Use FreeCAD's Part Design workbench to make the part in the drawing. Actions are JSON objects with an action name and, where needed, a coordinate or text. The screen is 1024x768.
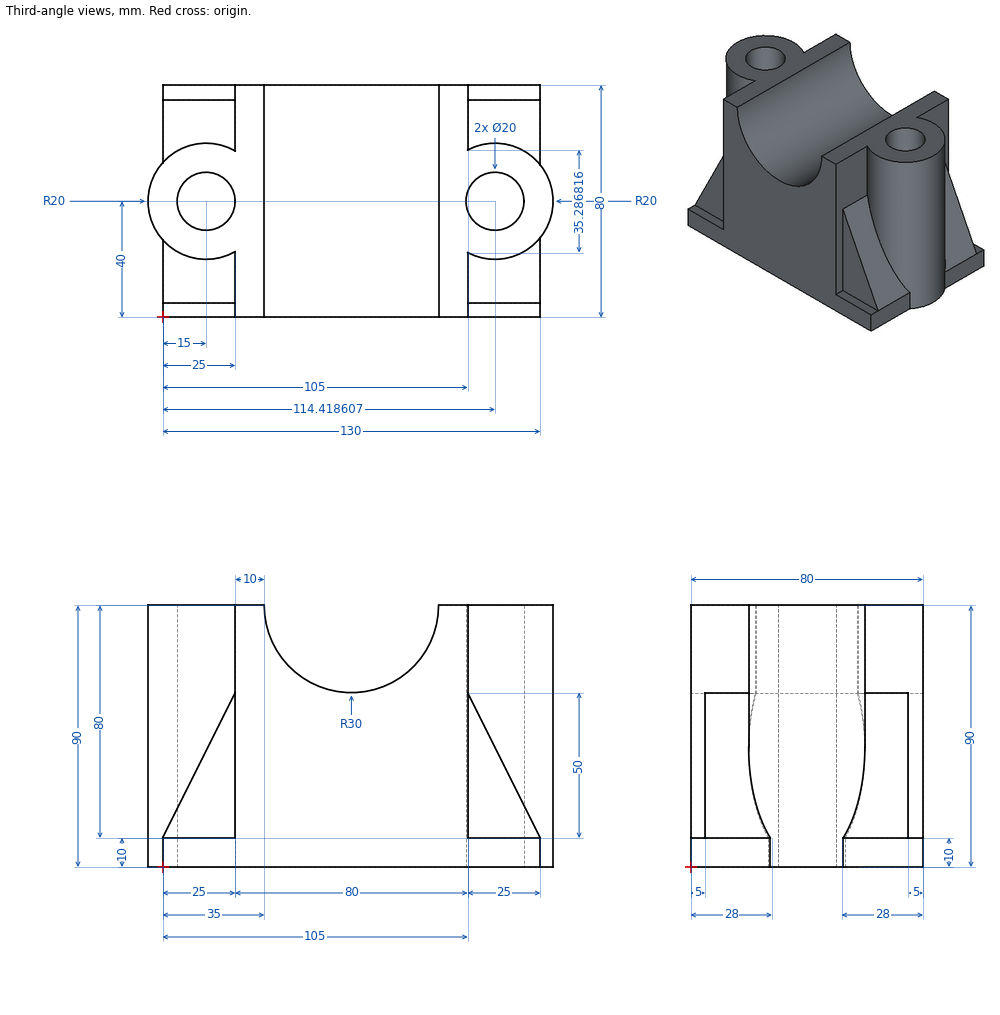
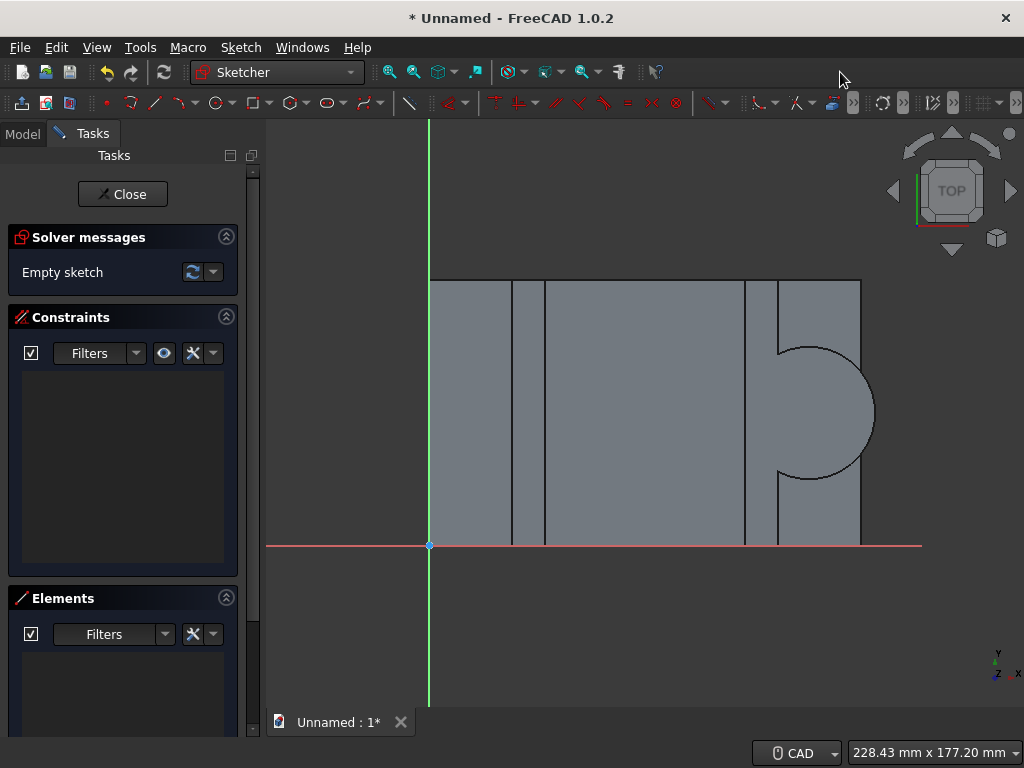
{"action": "scroll", "coordinate": [324, 496], "scroll_direction": "up", "scroll_amount": 3}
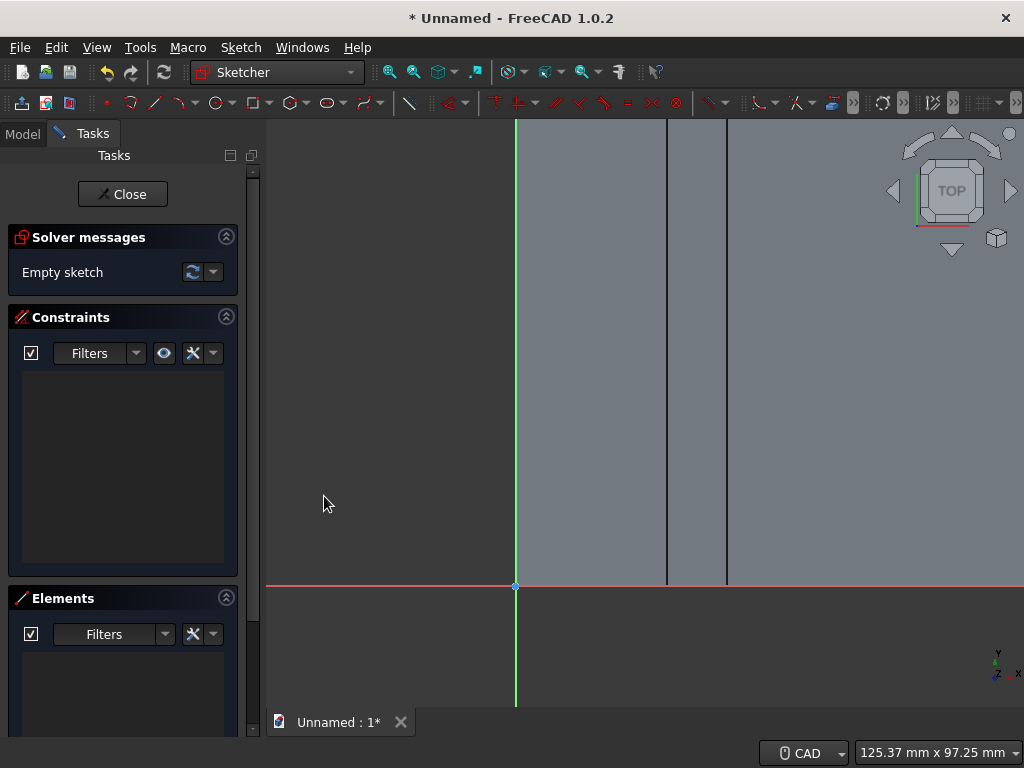
{"action": "left_click", "coordinate": [156, 104]}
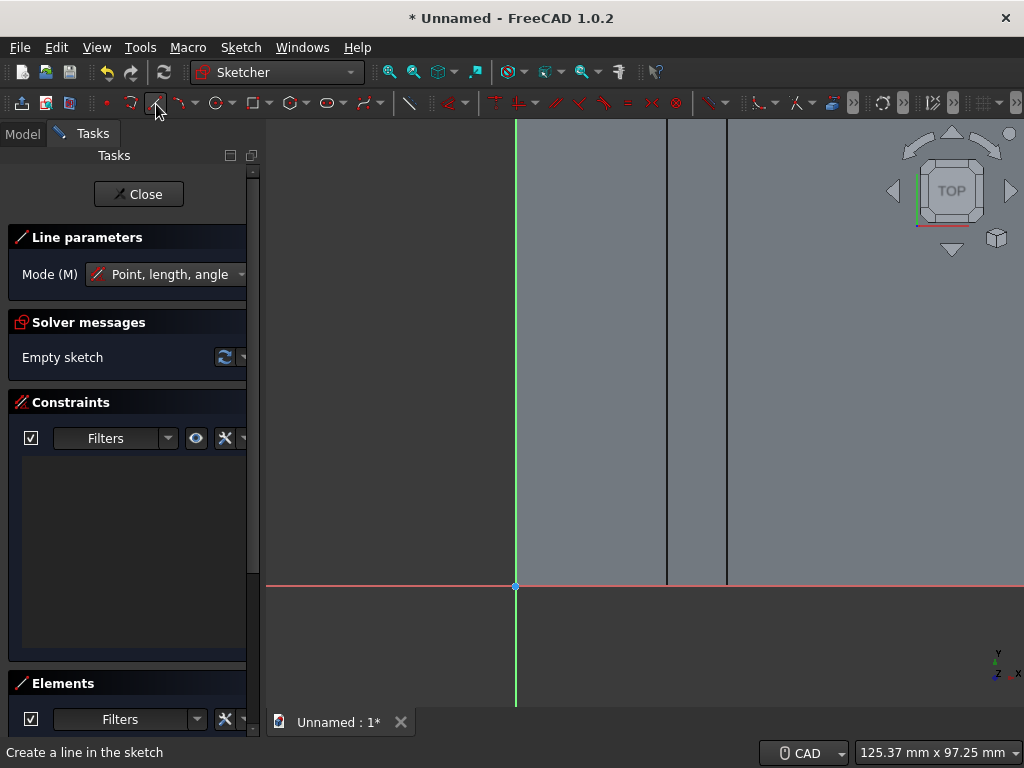
{"action": "left_click", "coordinate": [667, 449]}
{"action": "left_click", "coordinate": [667, 240]}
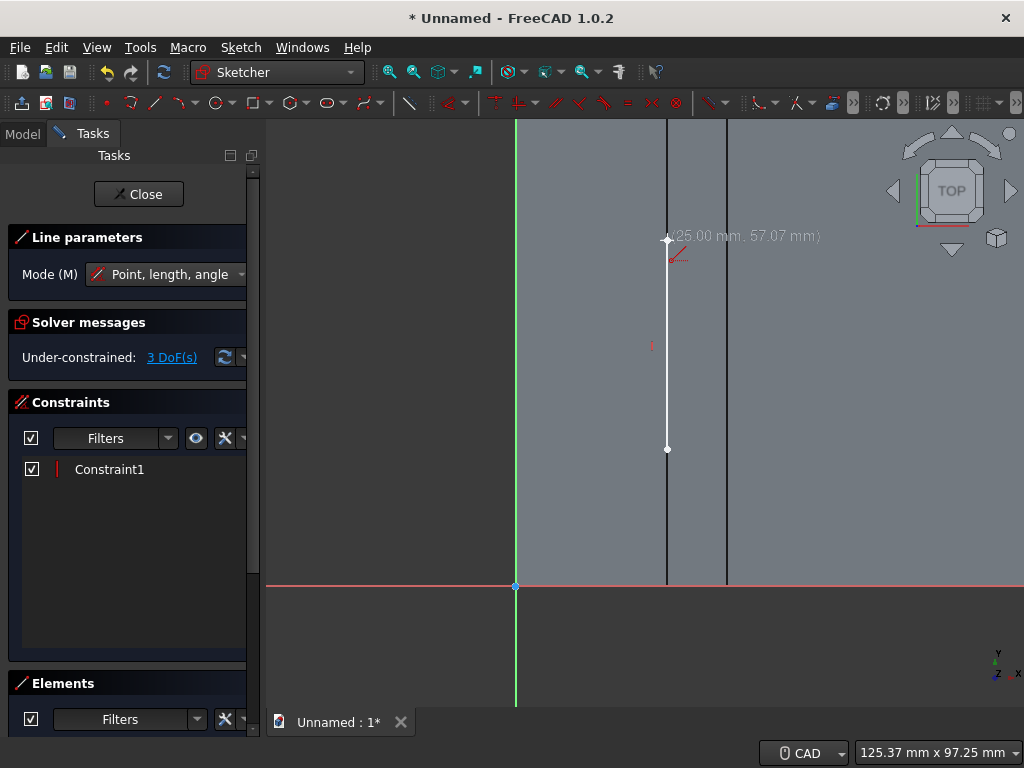
{"action": "left_click", "coordinate": [180, 104]}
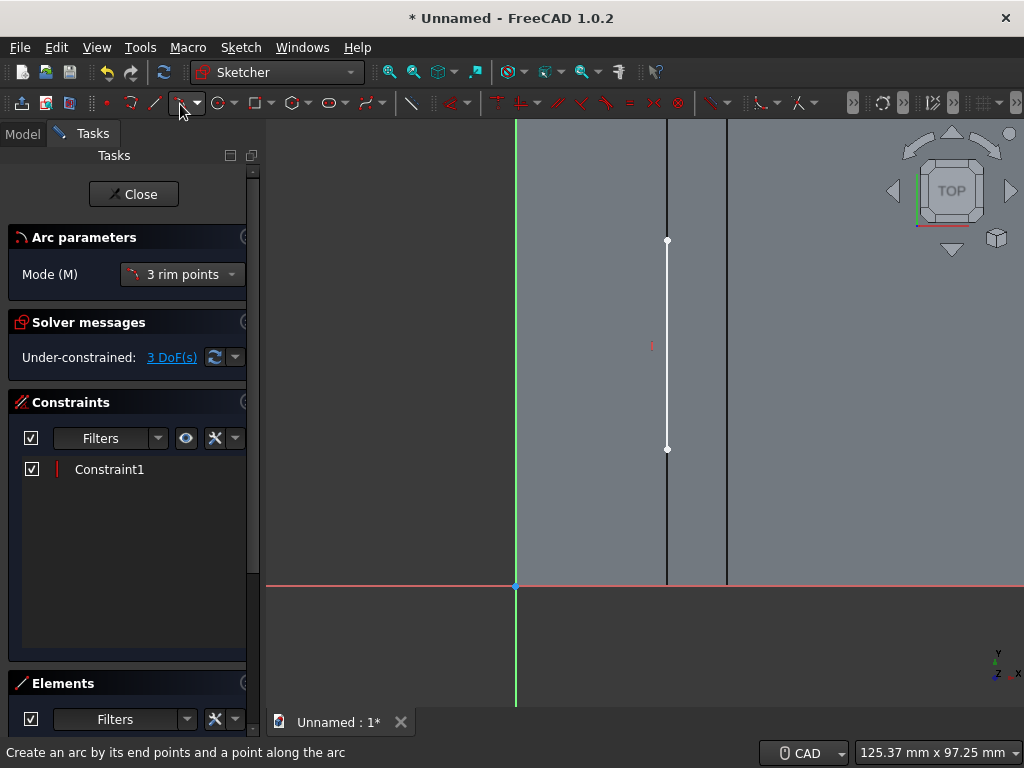
{"action": "left_click", "coordinate": [667, 241]}
{"action": "left_click", "coordinate": [667, 450]}
{"action": "left_click", "coordinate": [486, 344]}
{"action": "key", "text": "Escape"}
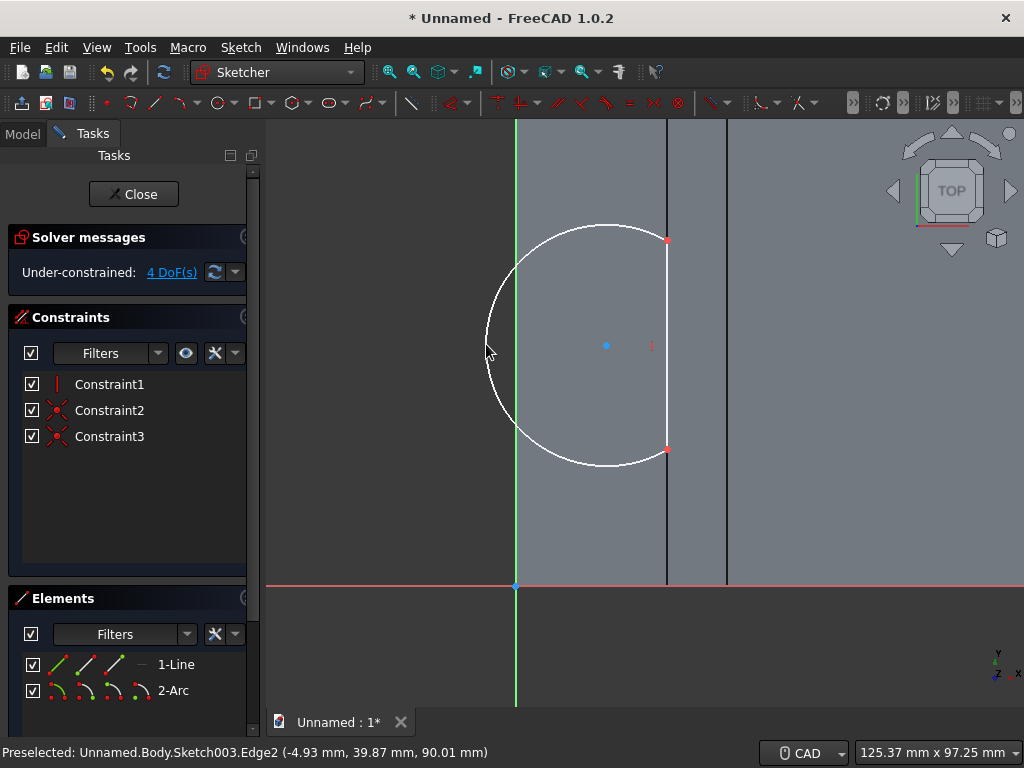
{"action": "left_click", "coordinate": [450, 104]}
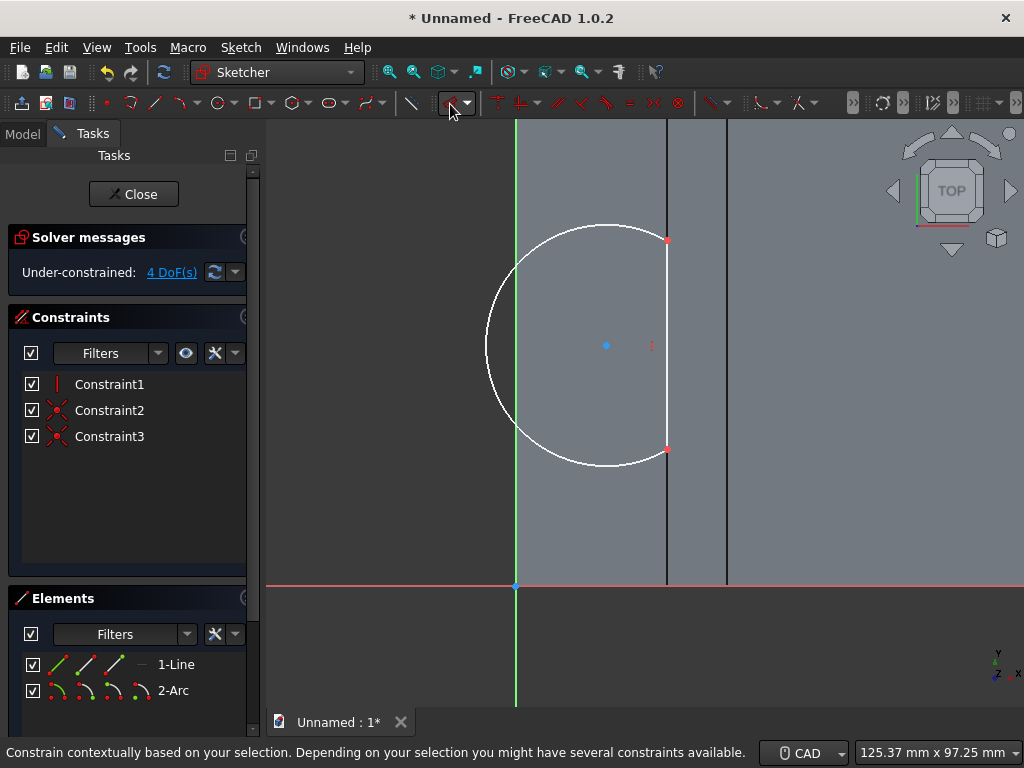
{"action": "scroll", "coordinate": [526, 256], "scroll_direction": "up", "scroll_amount": 2}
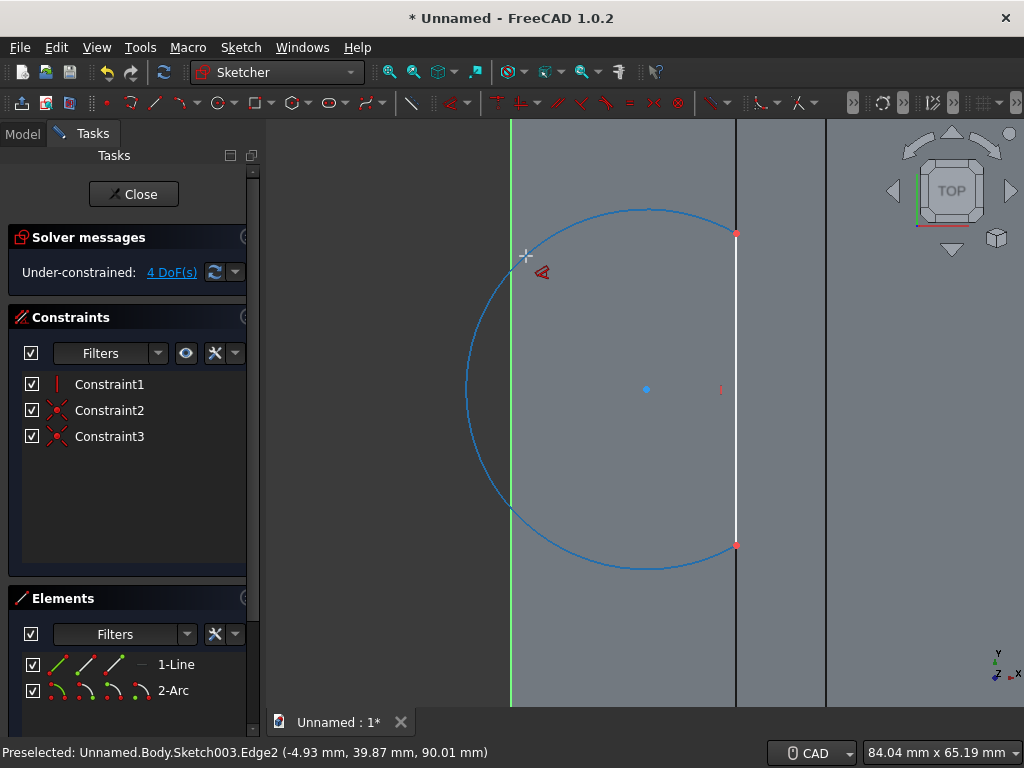
{"action": "left_click", "coordinate": [526, 256]}
{"action": "left_click", "coordinate": [597, 184]}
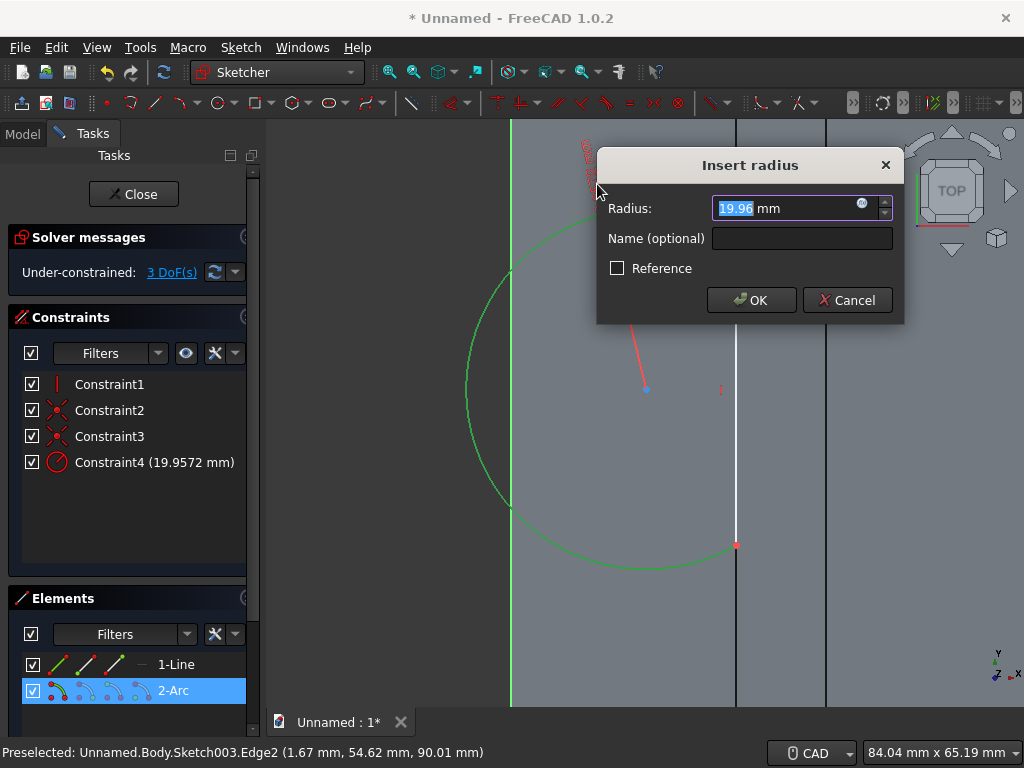
{"action": "type", "text": "20"}
{"action": "key", "text": "Return"}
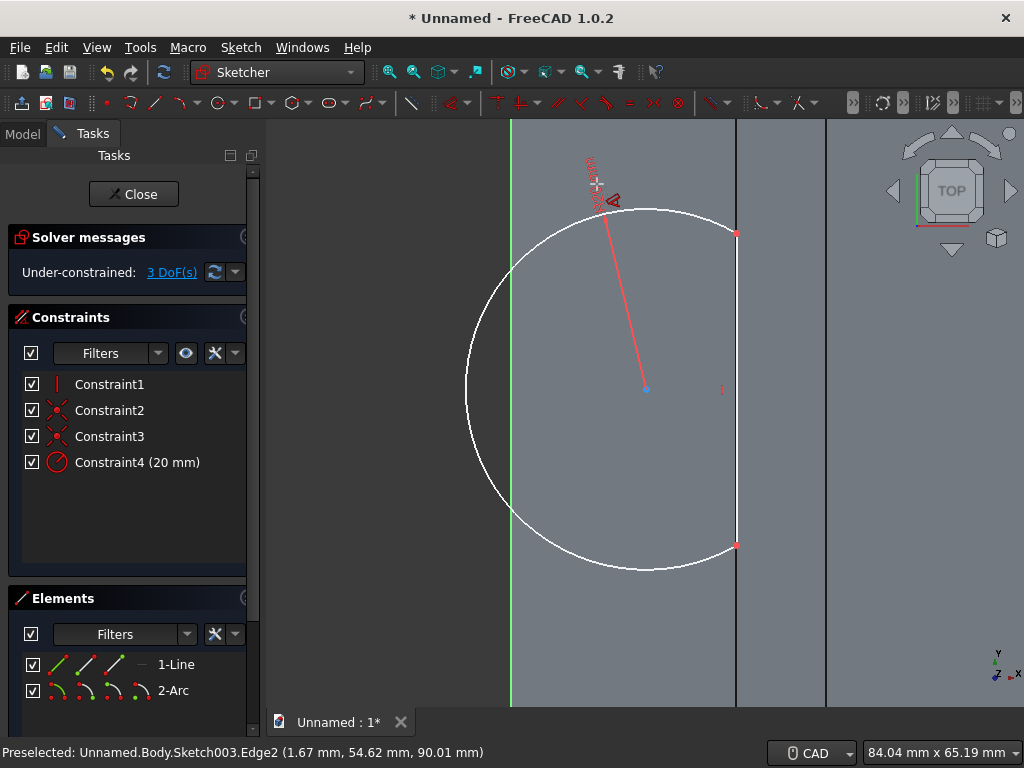
{"action": "left_click", "coordinate": [737, 545]}
{"action": "left_click", "coordinate": [624, 511]}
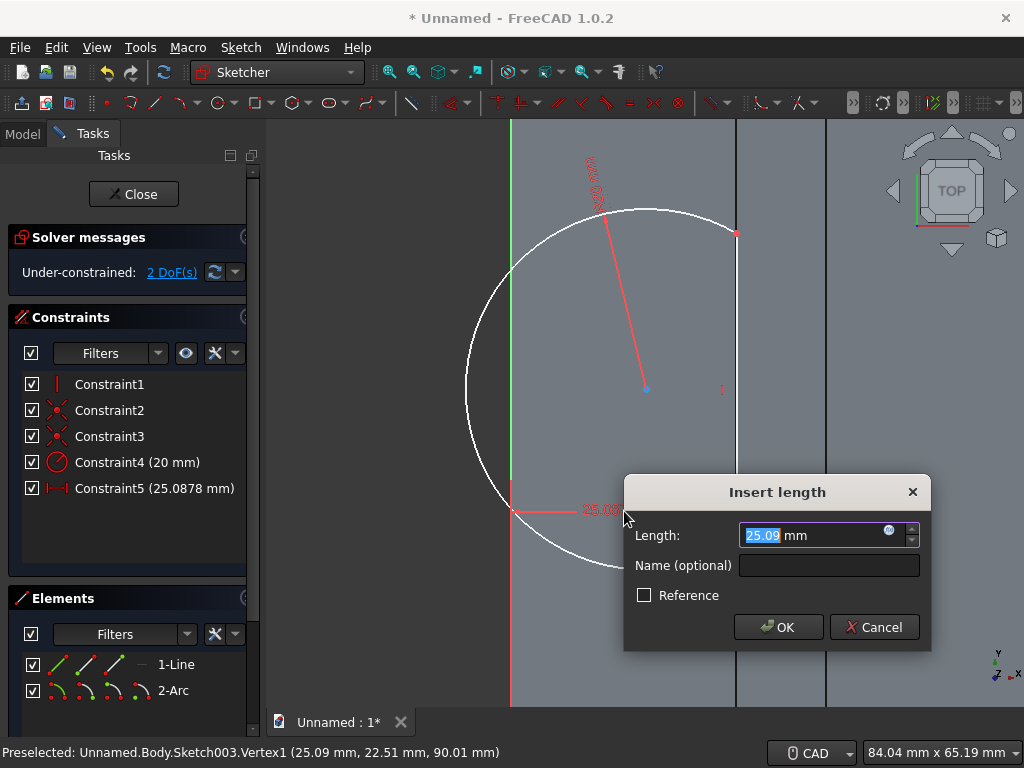
{"action": "type", "text": "25"}
{"action": "key", "text": "Return"}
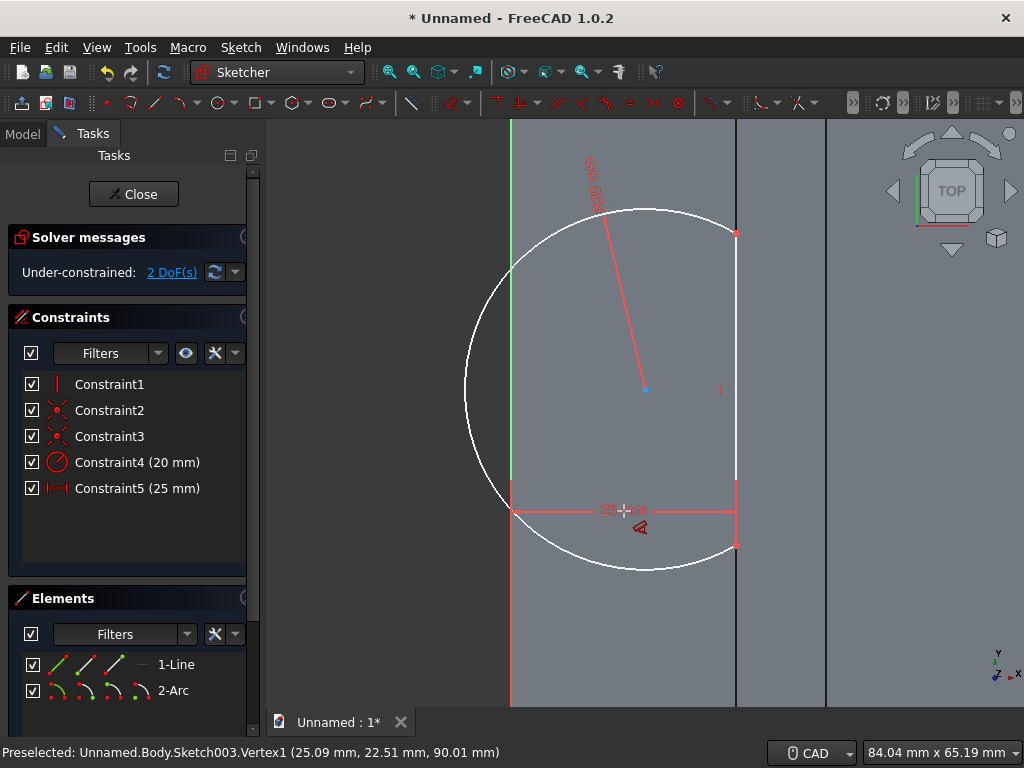
{"action": "left_click", "coordinate": [645, 389]}
{"action": "left_click", "coordinate": [578, 355]}